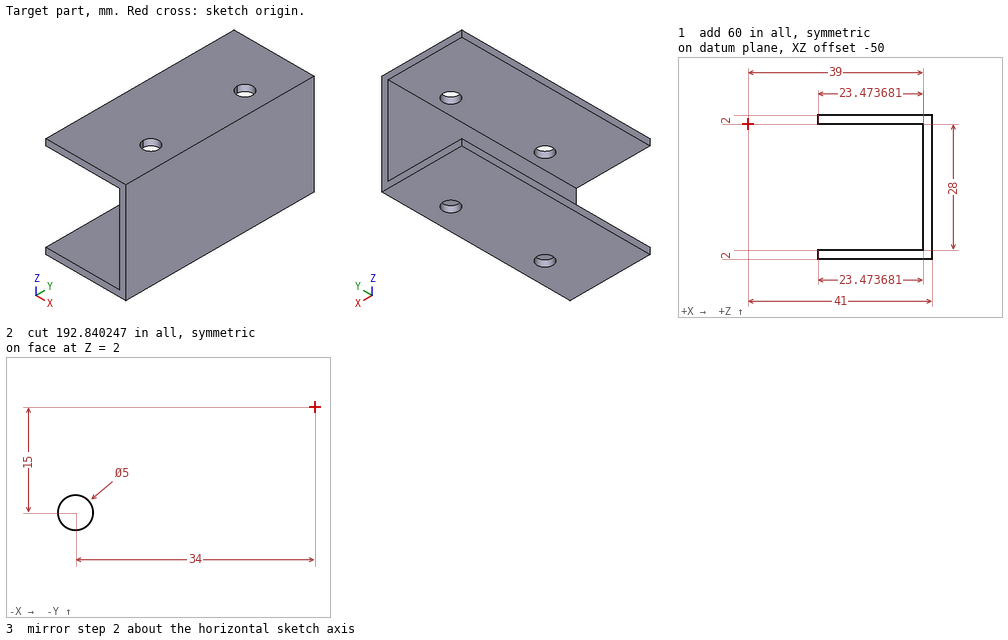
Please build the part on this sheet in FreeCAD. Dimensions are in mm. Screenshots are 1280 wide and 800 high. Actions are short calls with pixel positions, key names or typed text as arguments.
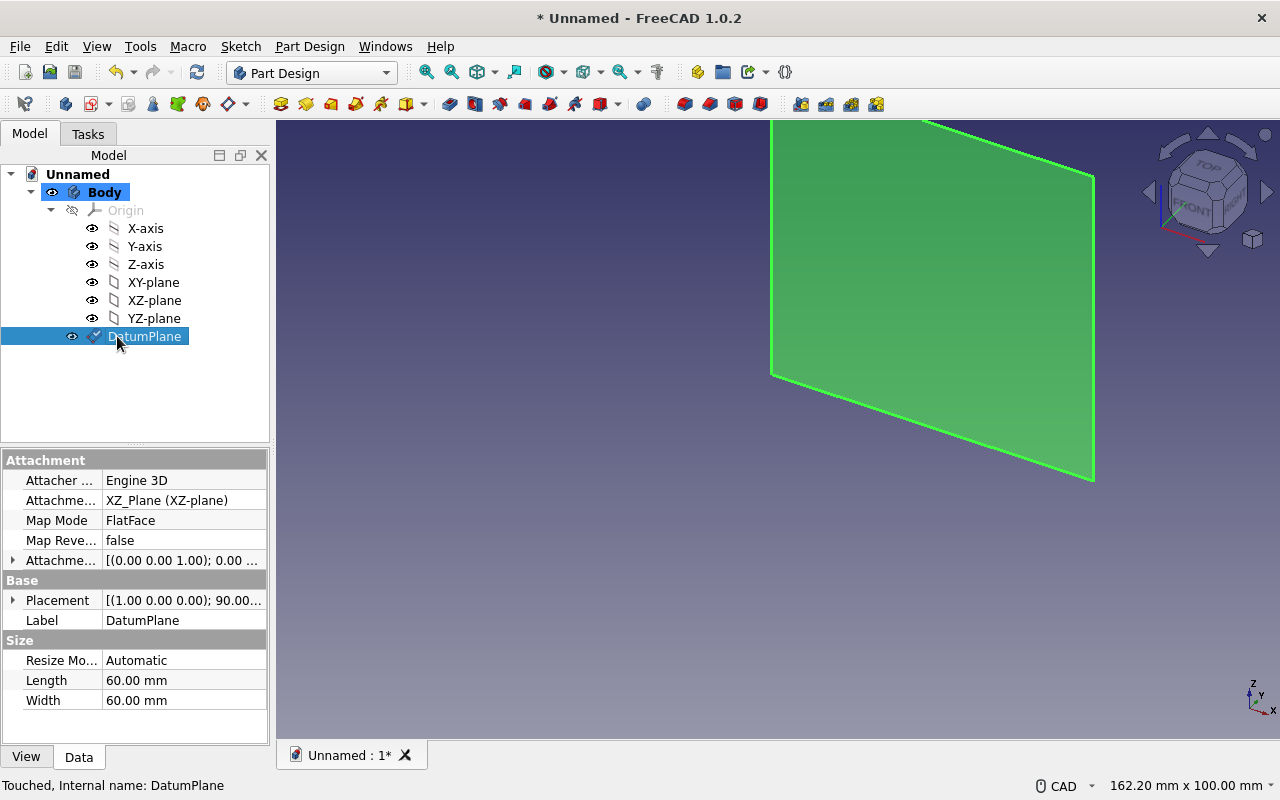
click(90, 104)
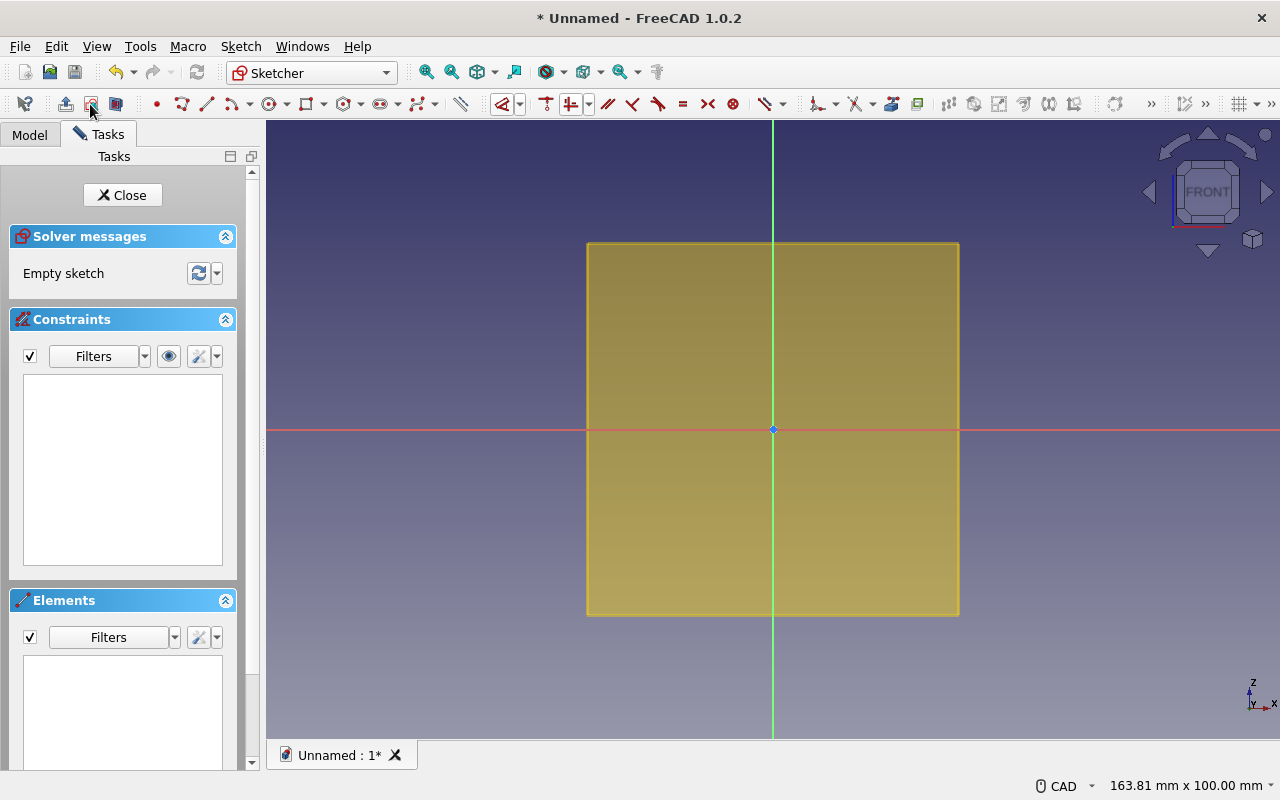
scroll(1115, 622, up, 3)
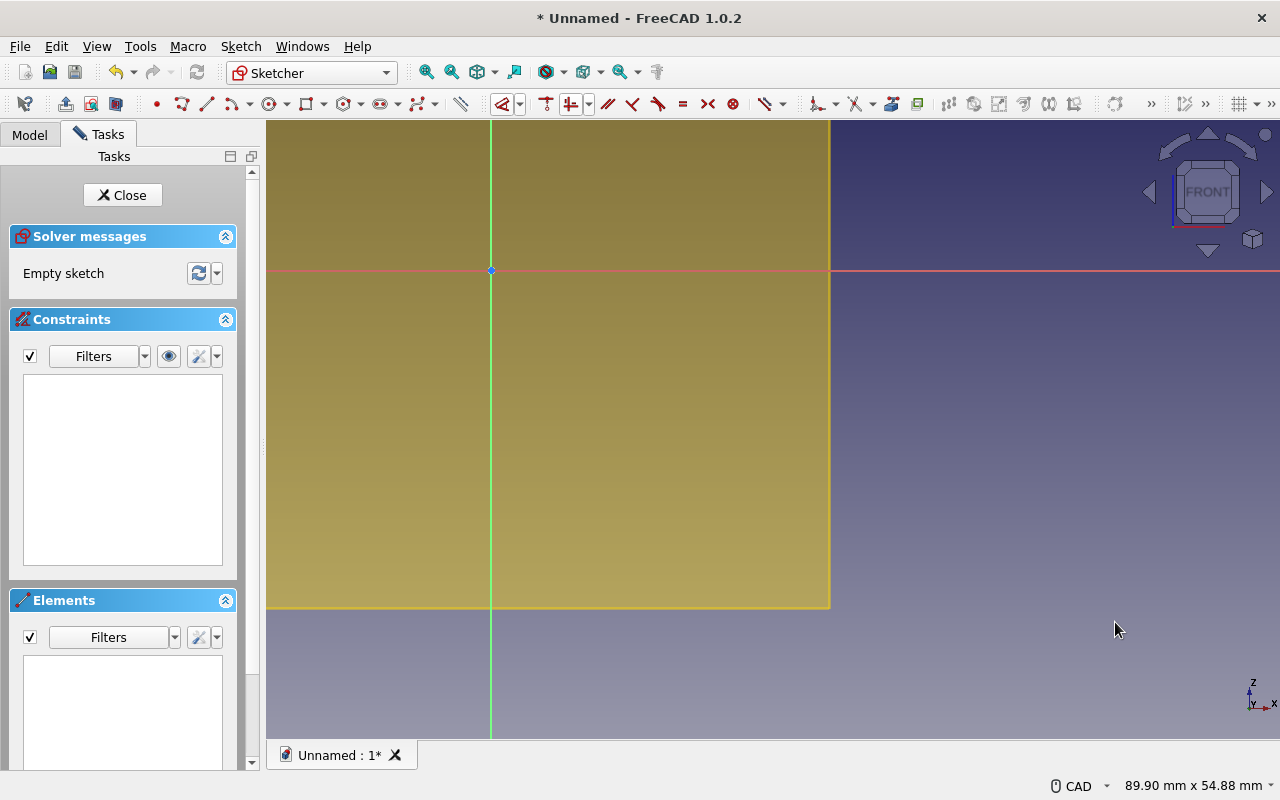
click(182, 104)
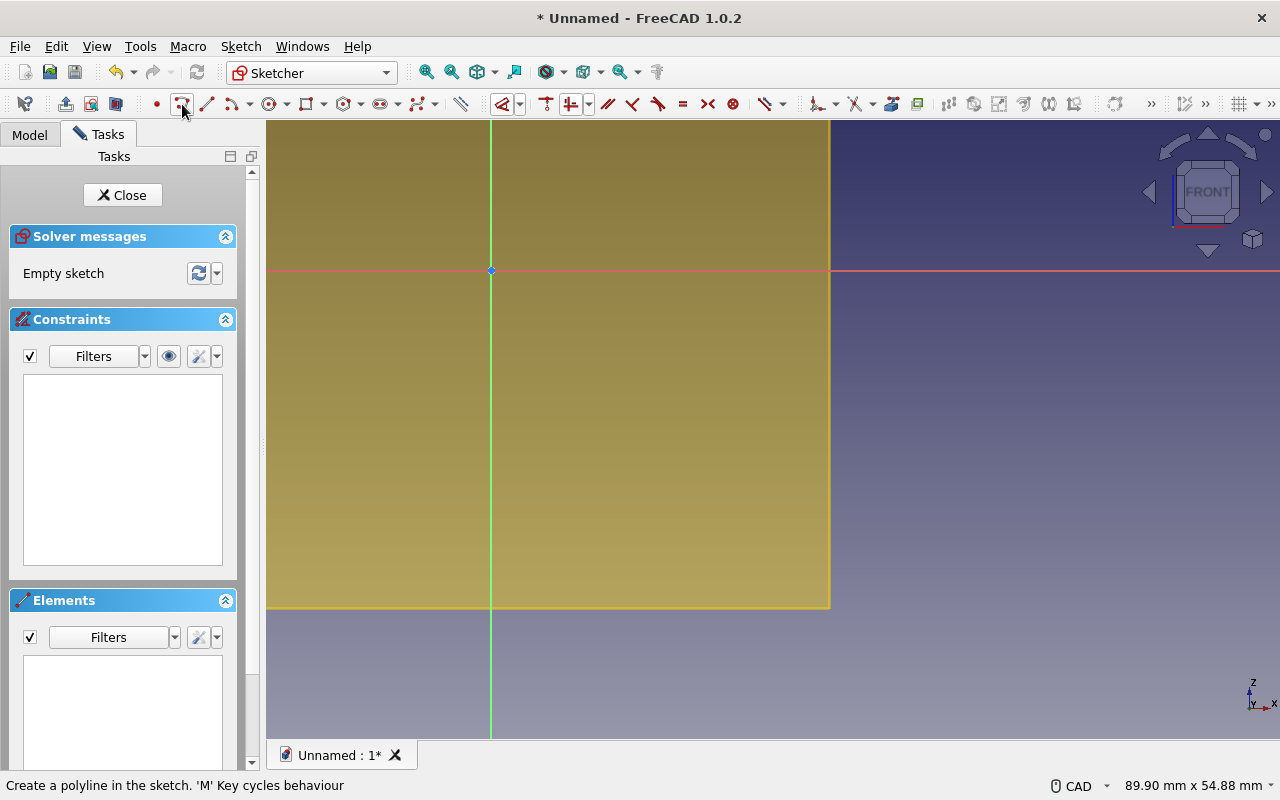
click(666, 271)
click(931, 280)
click(931, 586)
click(666, 586)
click(666, 609)
click(954, 609)
click(954, 248)
click(666, 248)
click(666, 271)
key(Escape)
key(Escape)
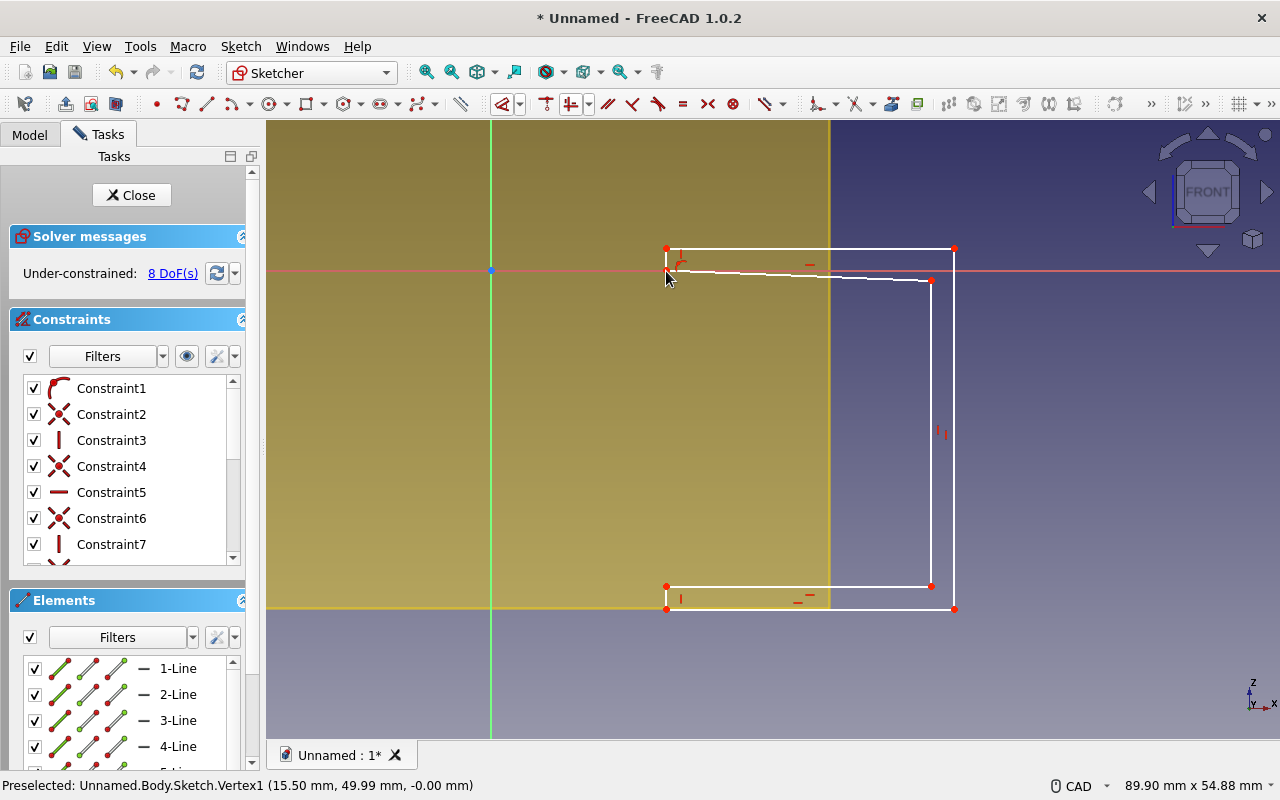
click(745, 274)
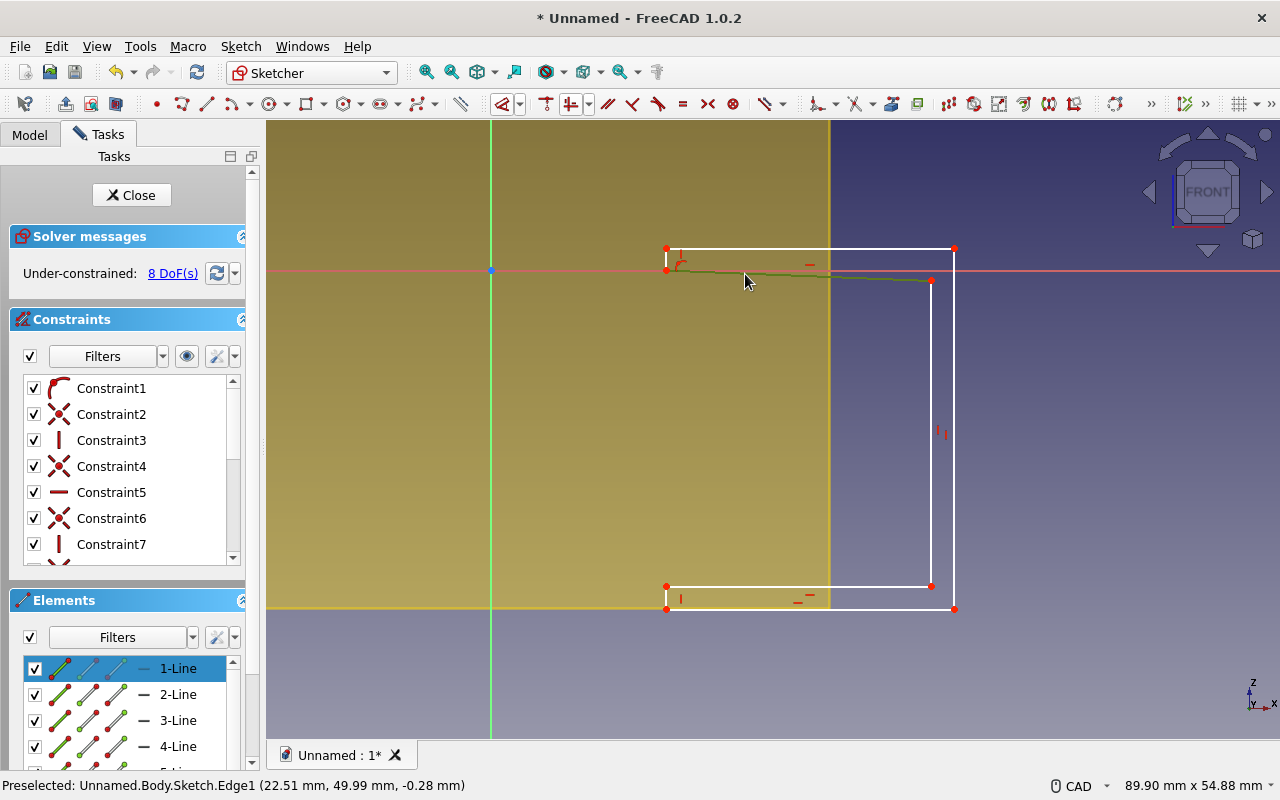
click(588, 104)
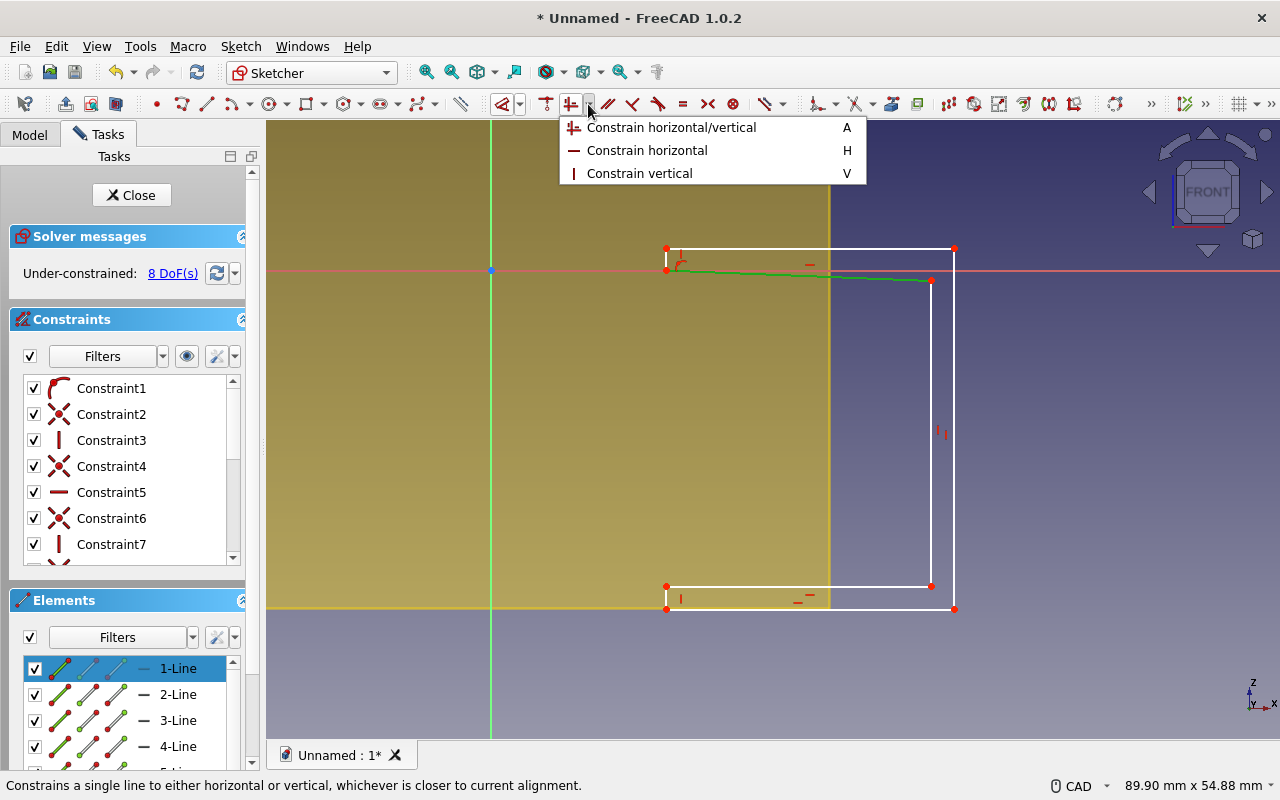
click(713, 150)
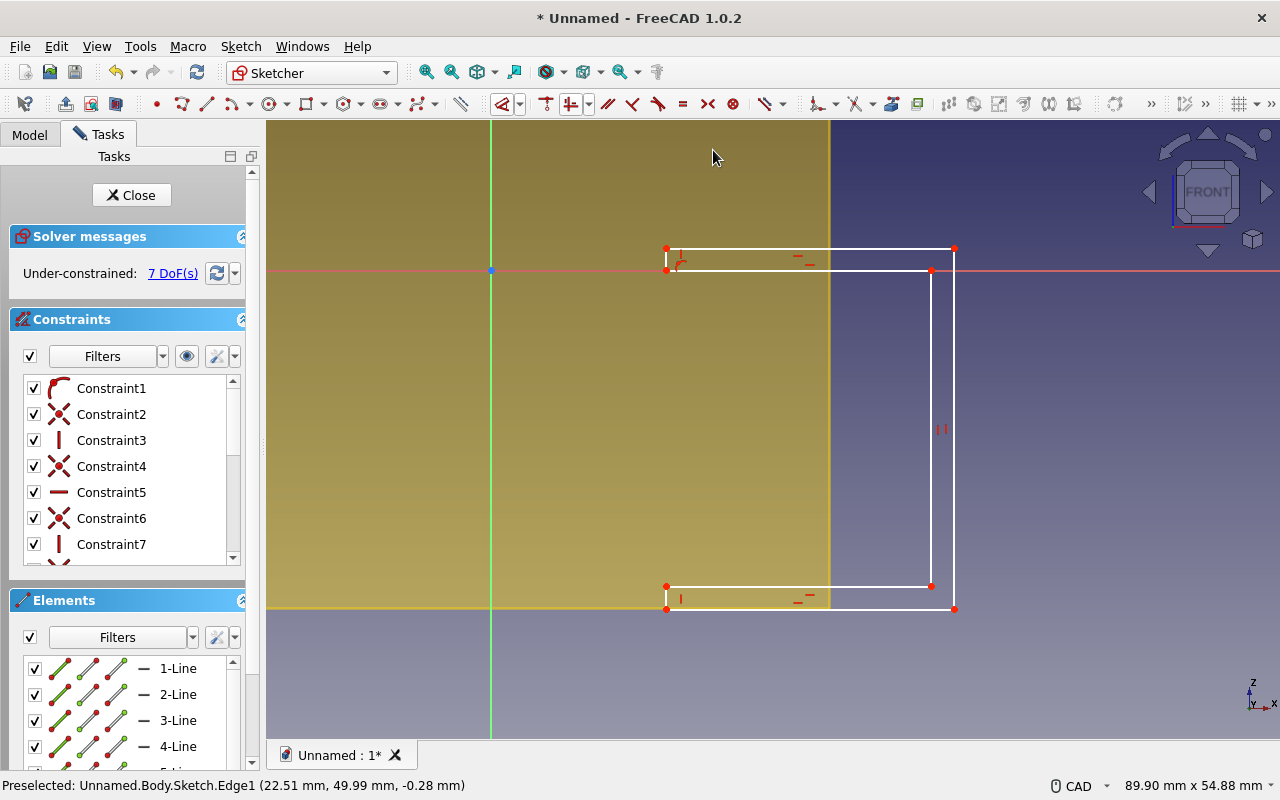
click(502, 104)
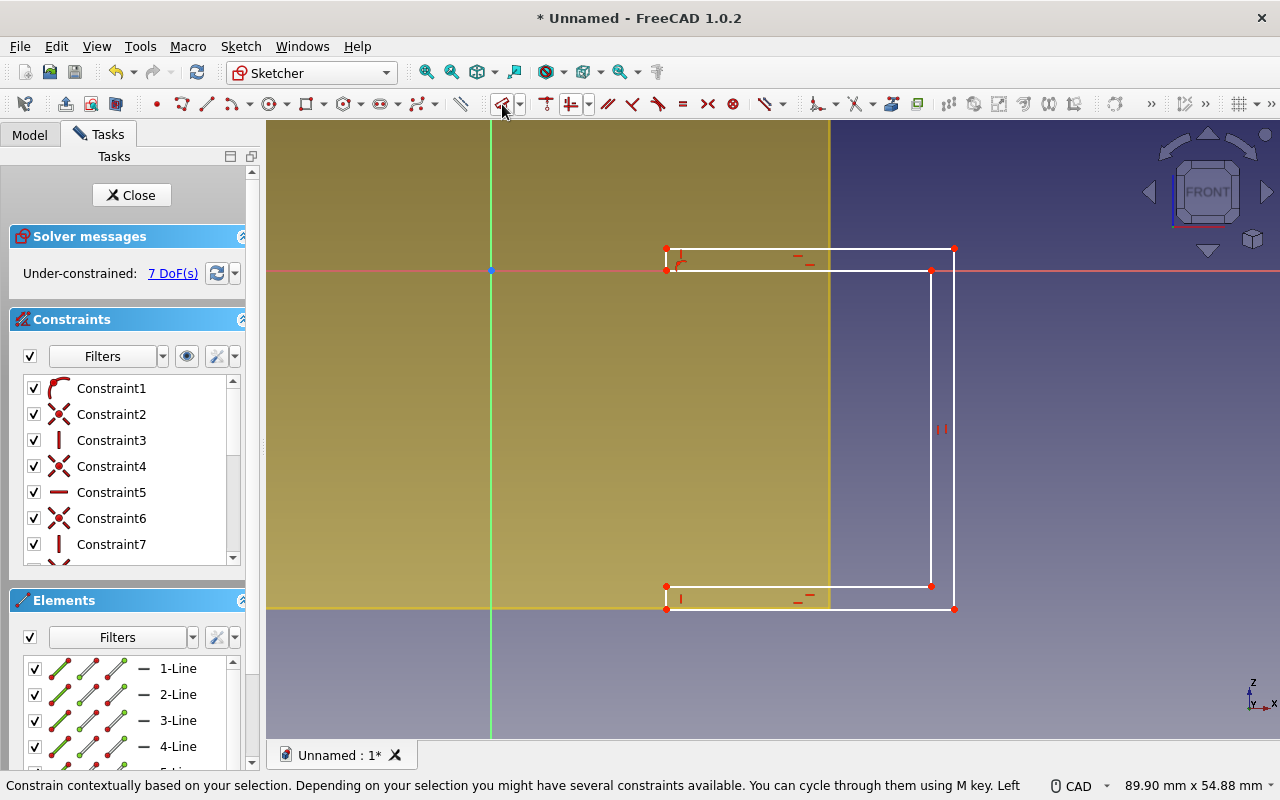
scroll(666, 596, up, 3)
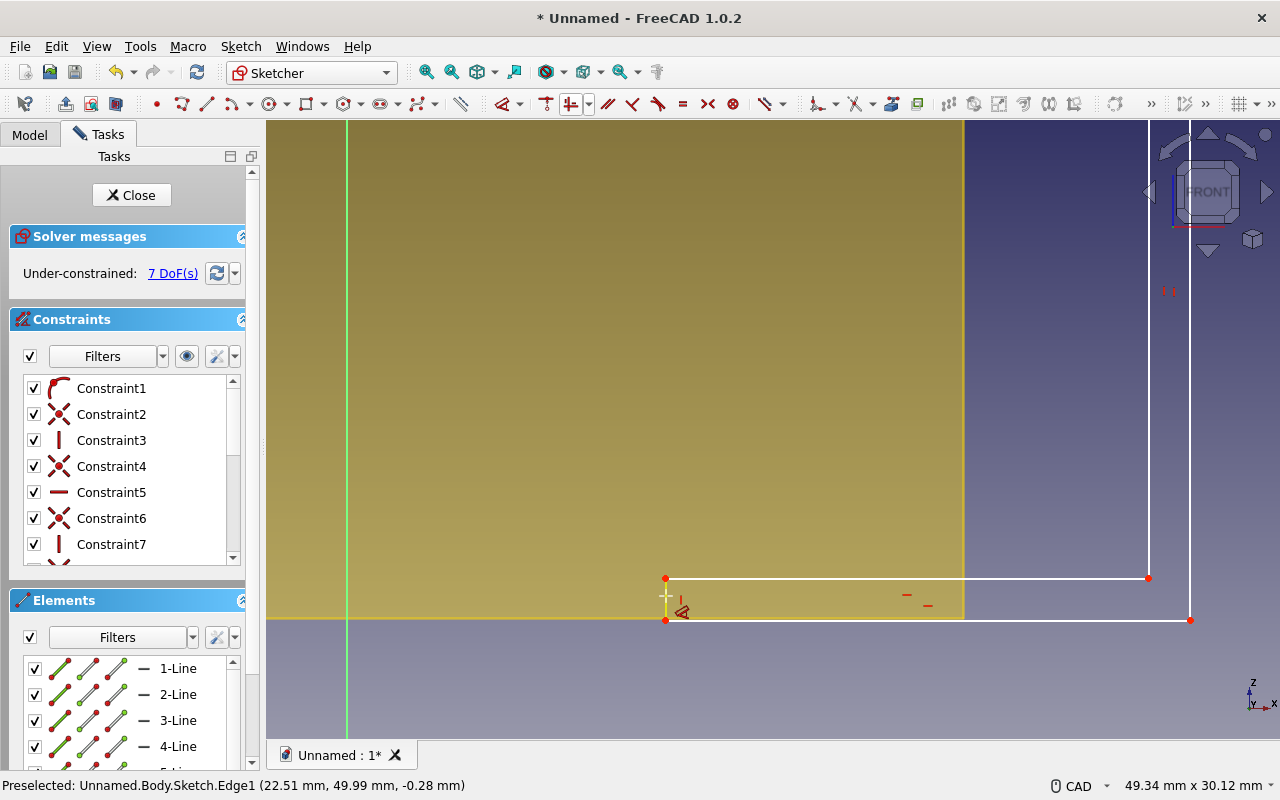
click(666, 596)
click(632, 600)